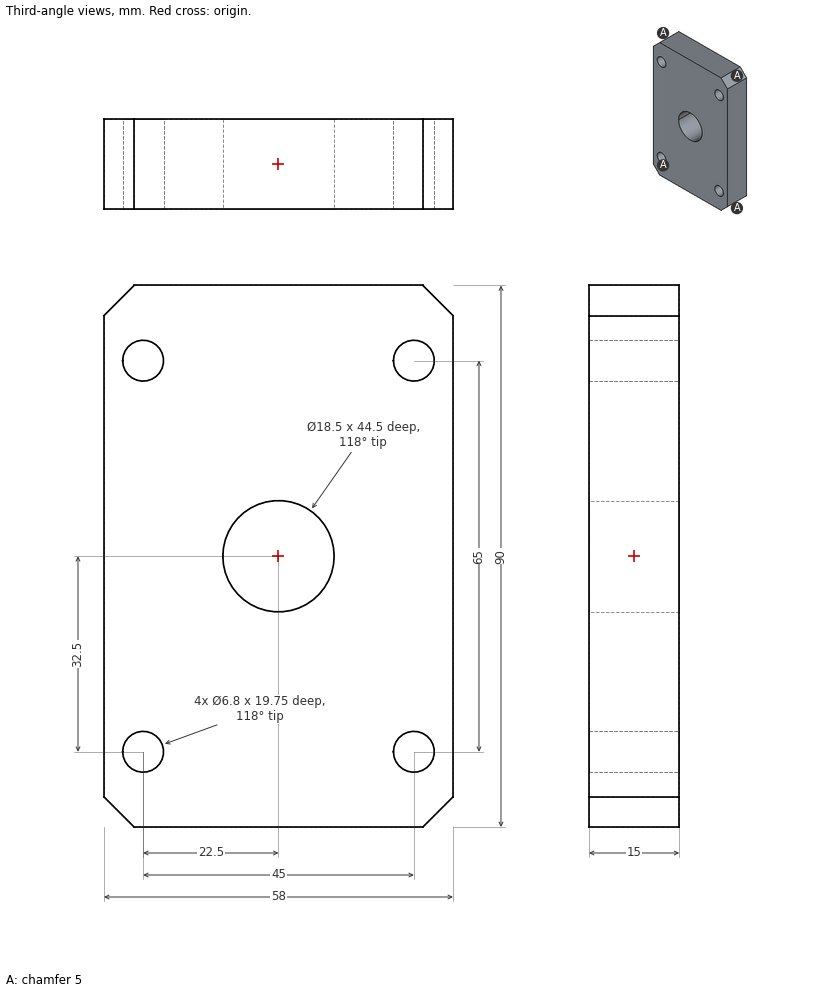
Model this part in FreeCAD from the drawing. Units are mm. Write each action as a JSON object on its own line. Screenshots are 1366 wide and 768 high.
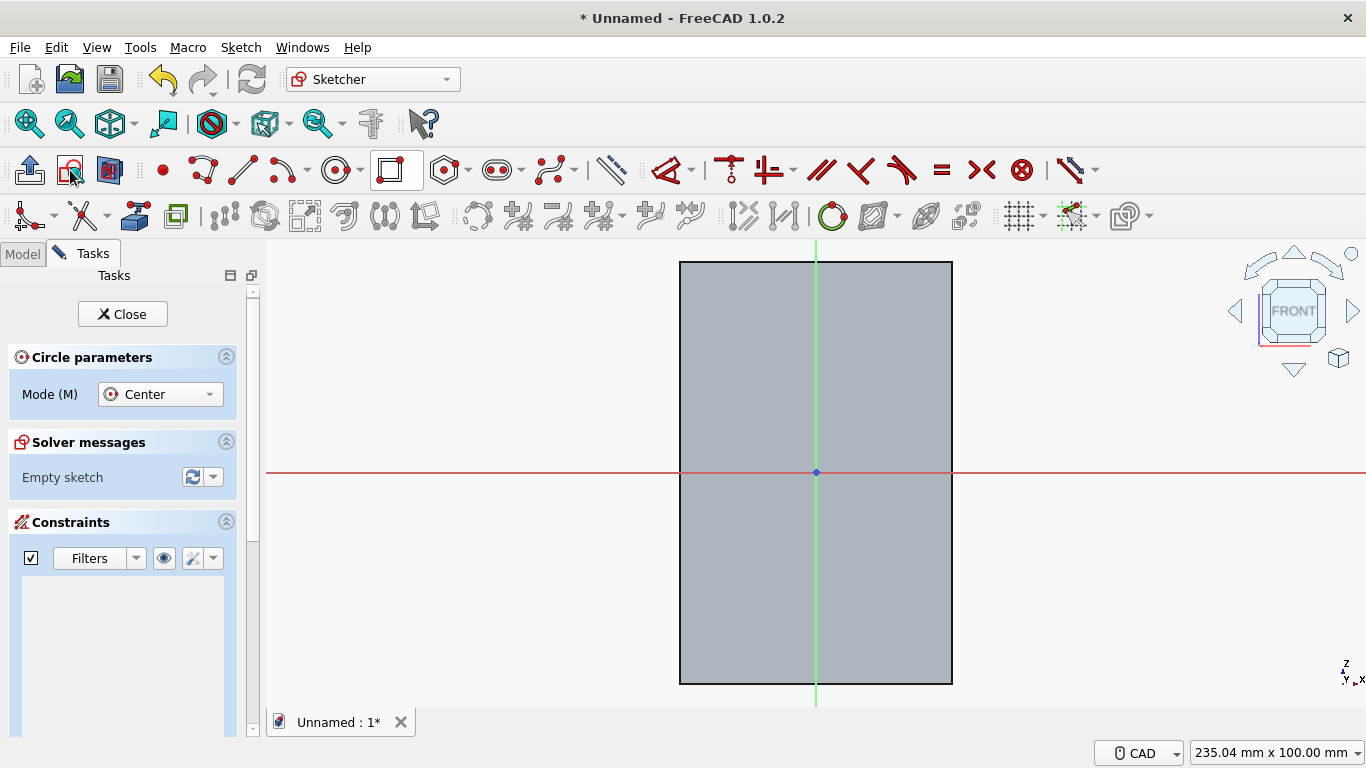
{"action": "scroll", "coordinate": [711, 625], "scroll_direction": "up", "scroll_amount": 2}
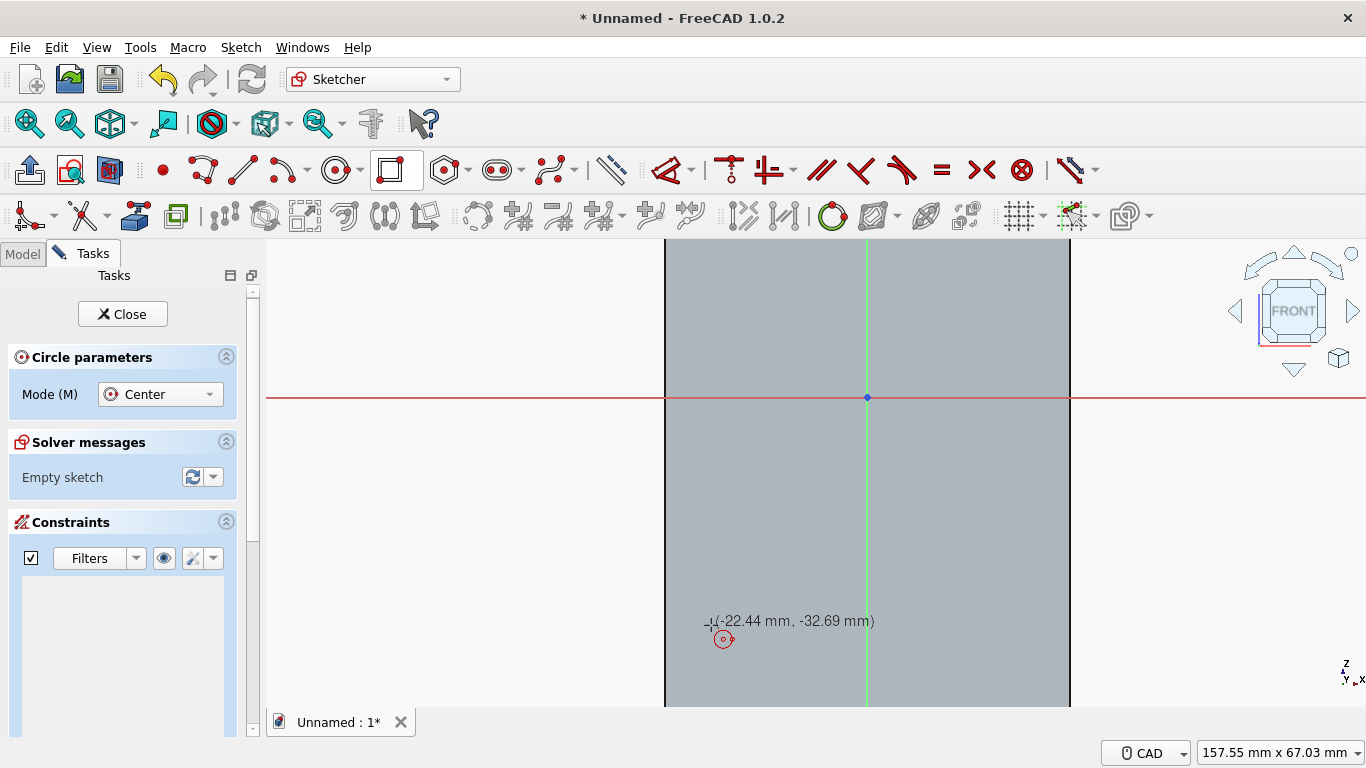
{"action": "left_click", "coordinate": [710, 625]}
{"action": "left_click", "coordinate": [727, 608]}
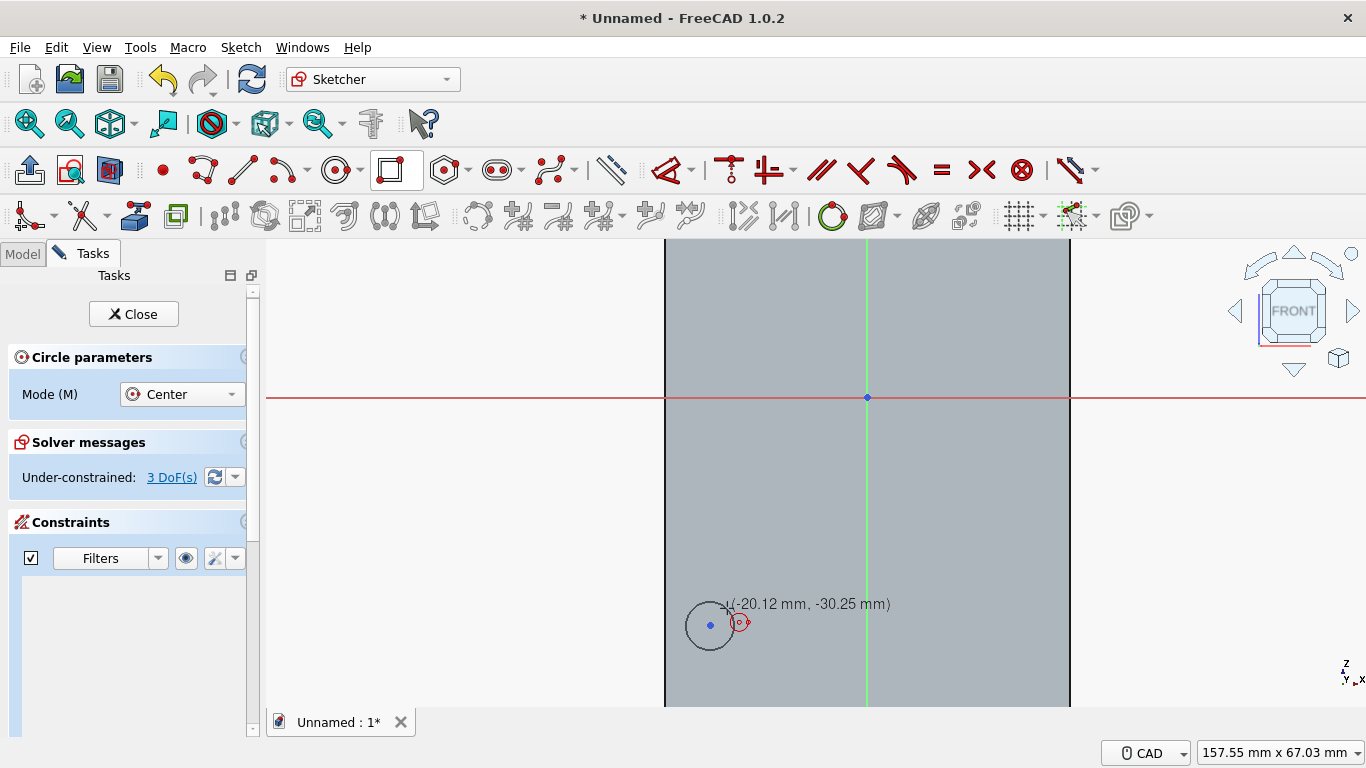
{"action": "left_click", "coordinate": [1025, 625]}
{"action": "left_click", "coordinate": [1041, 608]}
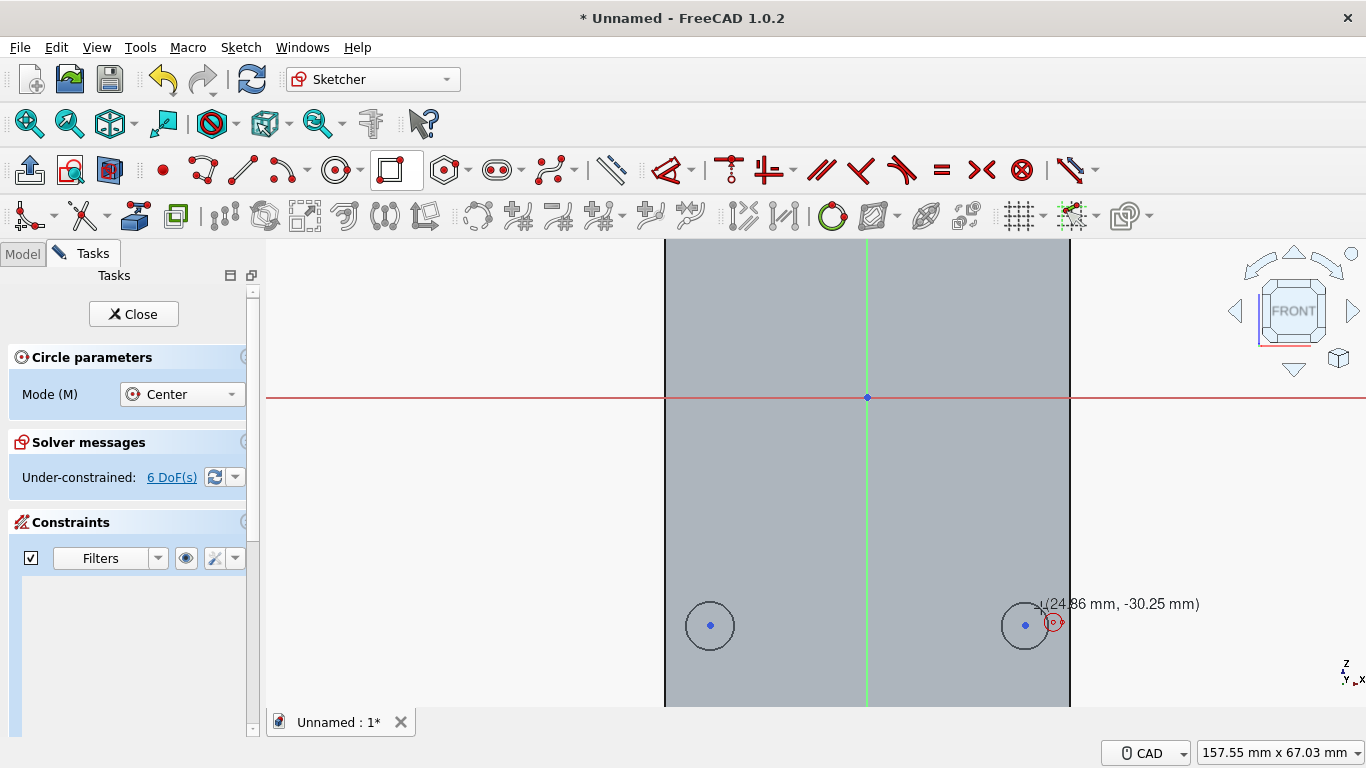
{"action": "scroll", "coordinate": [602, 564], "scroll_direction": "down", "scroll_amount": 3}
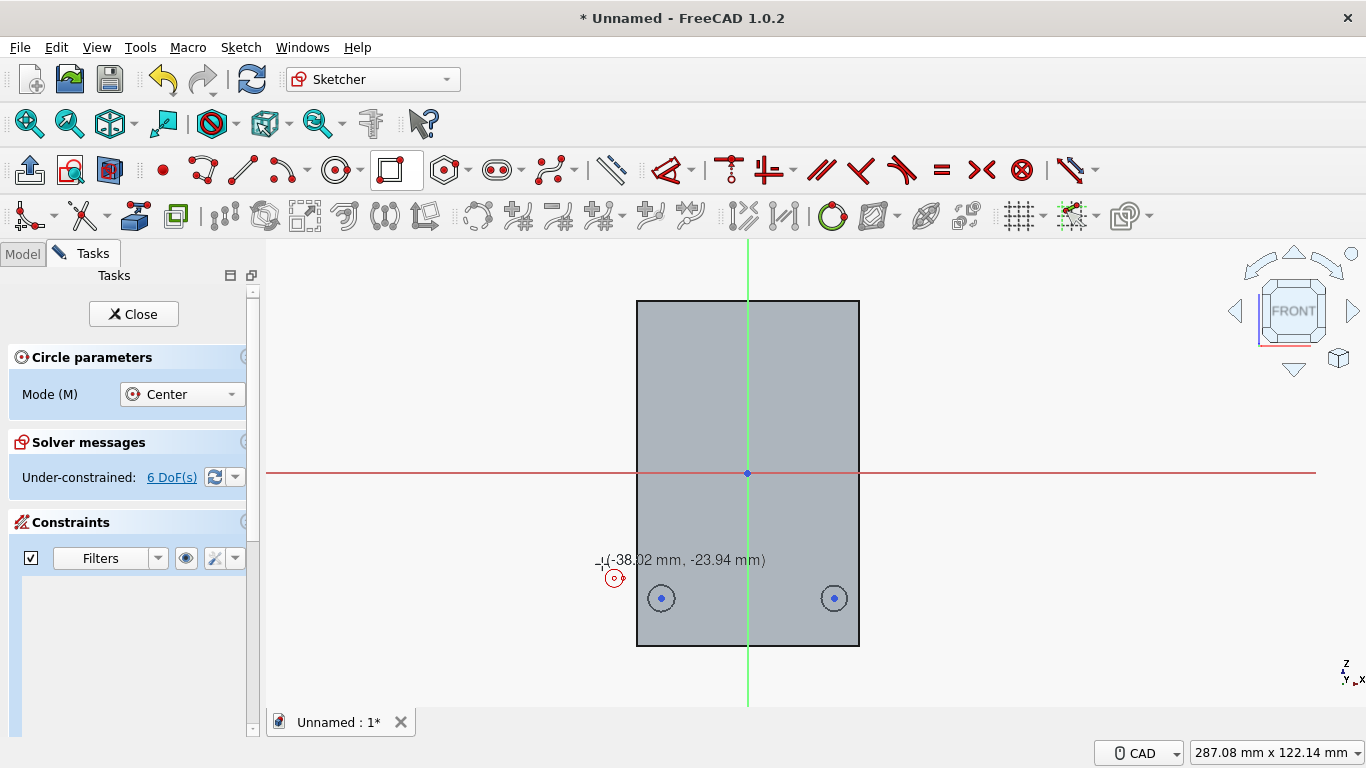
{"action": "scroll", "coordinate": [834, 349], "scroll_direction": "up", "scroll_amount": 3}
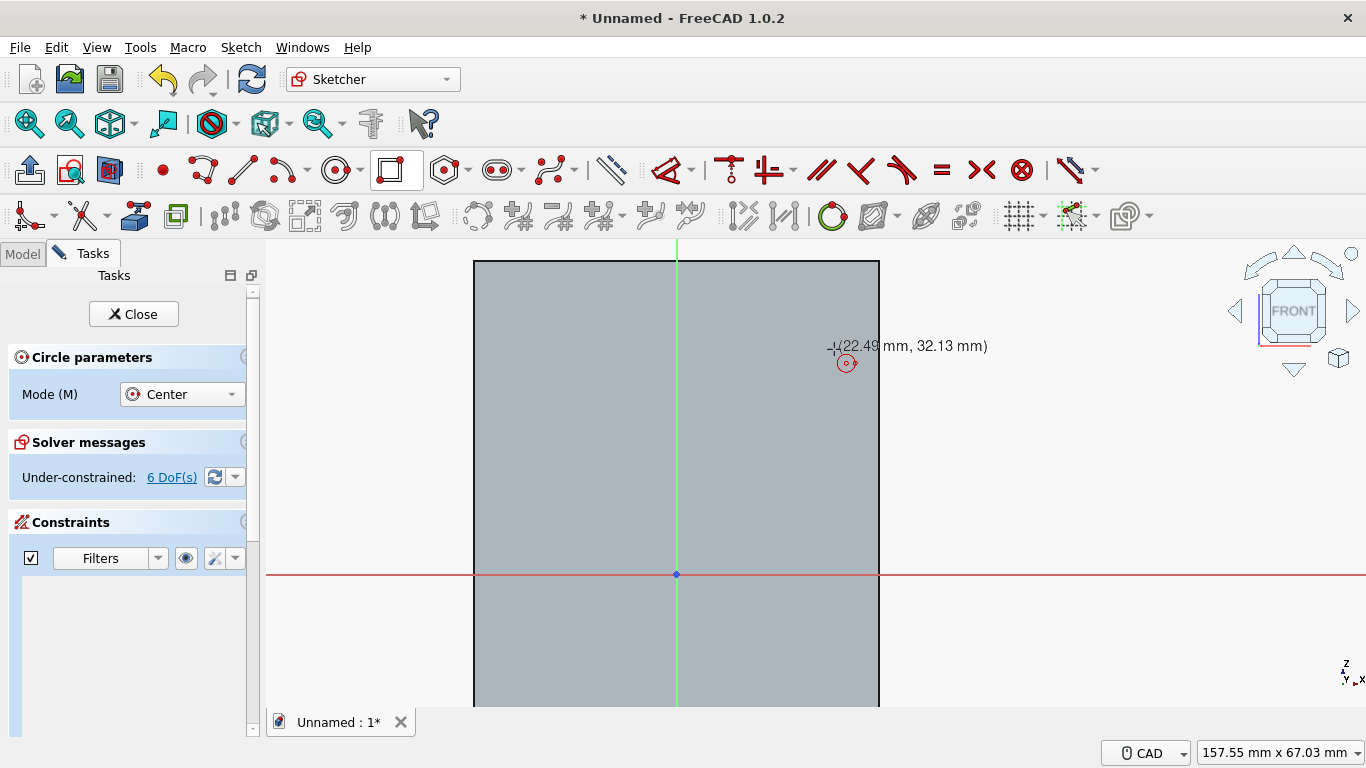
{"action": "left_click", "coordinate": [834, 348]}
{"action": "left_click", "coordinate": [850, 331]}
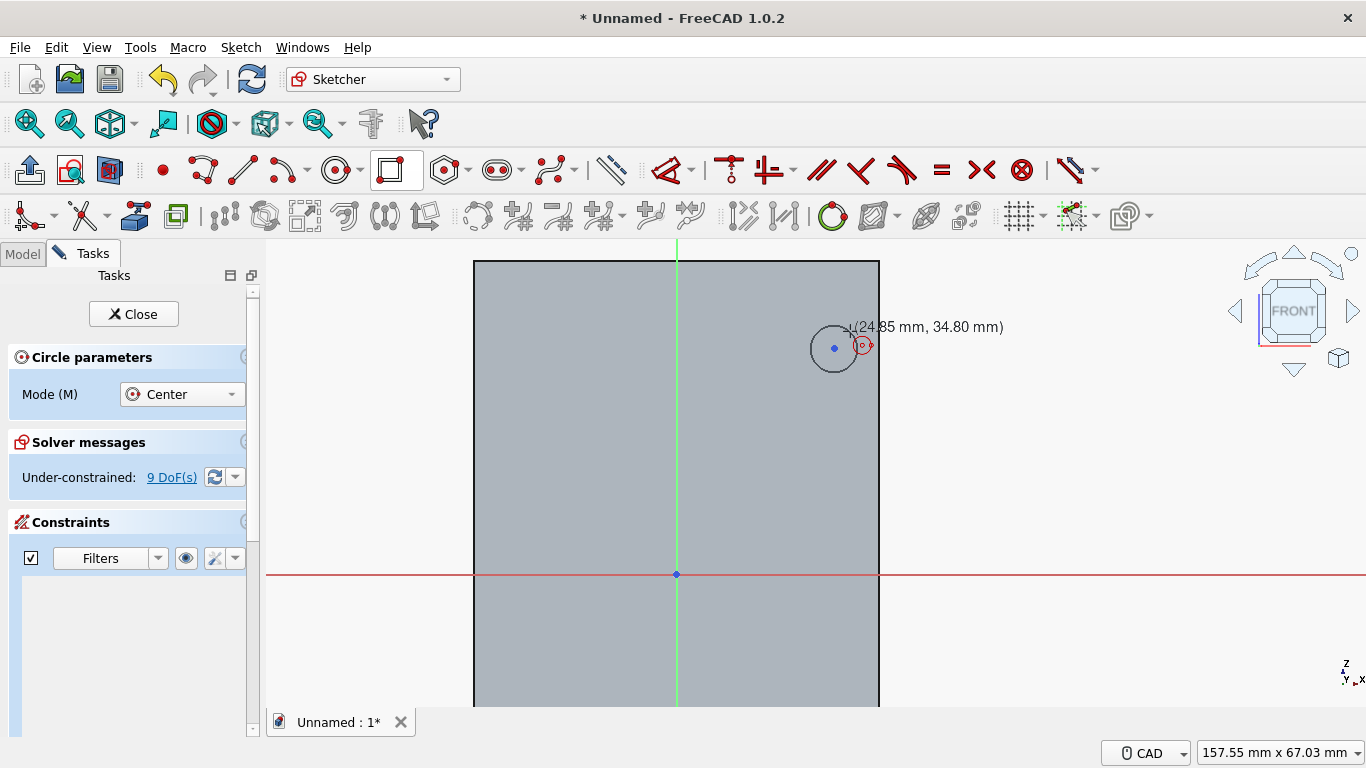
{"action": "left_click", "coordinate": [519, 348]}
{"action": "left_click", "coordinate": [536, 331]}
{"action": "key", "text": "Escape"}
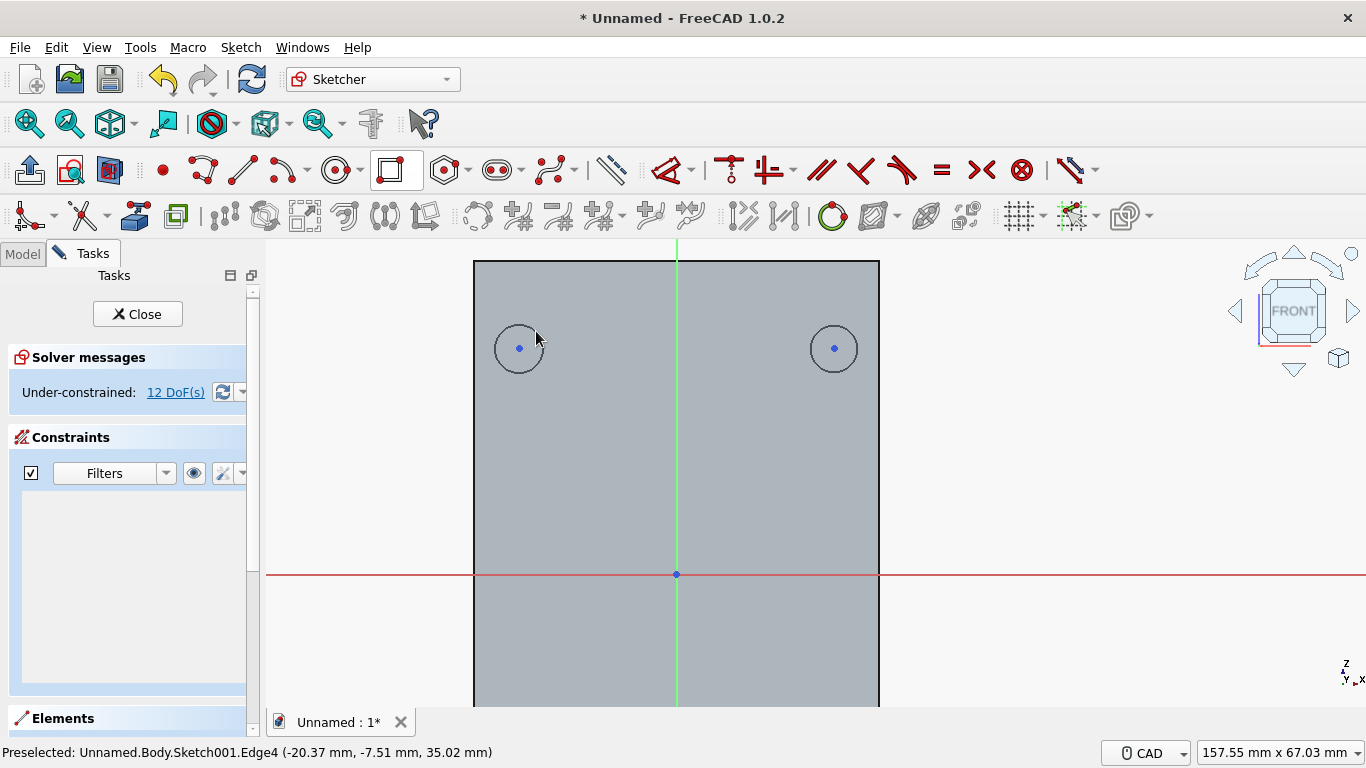
{"action": "scroll", "coordinate": [834, 349], "scroll_direction": "down", "scroll_amount": 3}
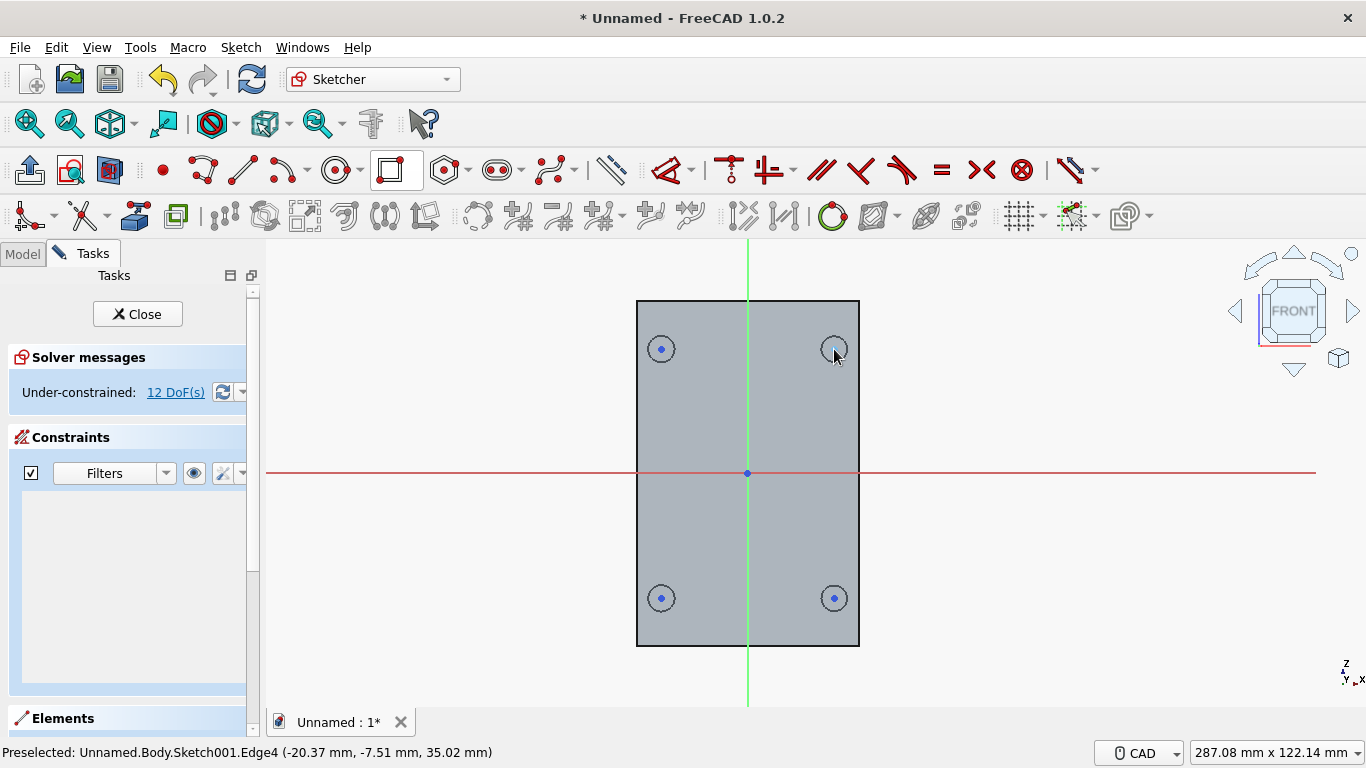
{"action": "left_click", "coordinate": [671, 589]}